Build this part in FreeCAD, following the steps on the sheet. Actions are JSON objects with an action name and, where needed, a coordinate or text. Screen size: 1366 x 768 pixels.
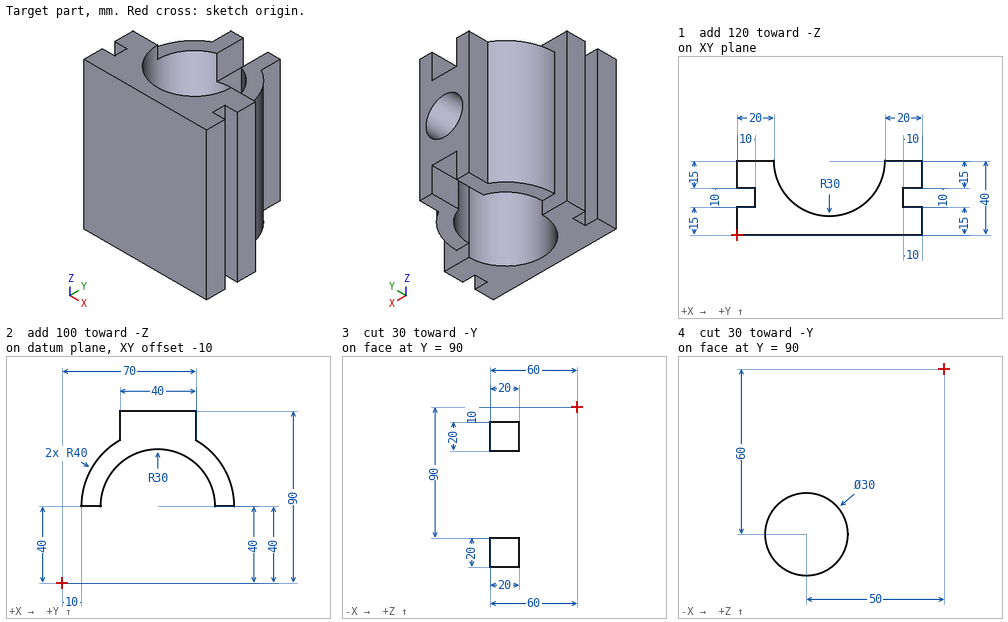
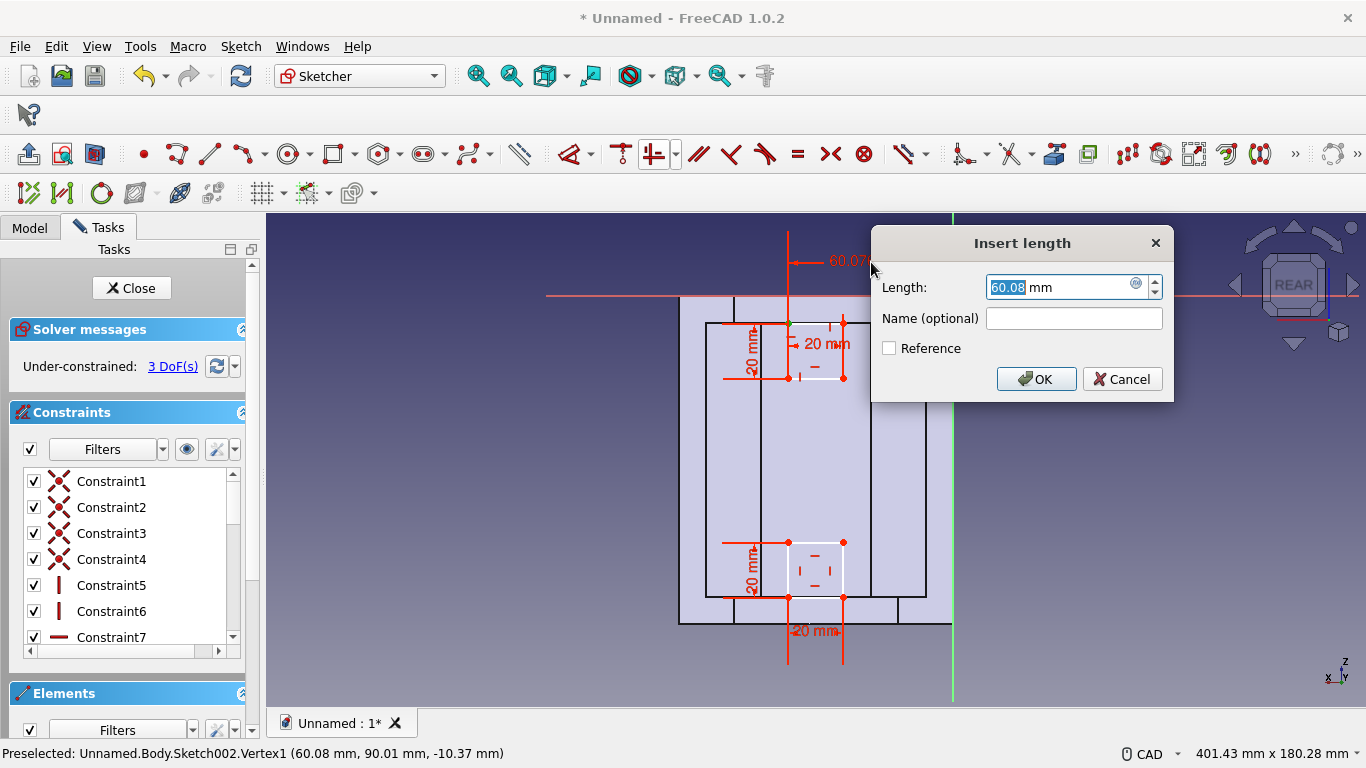
{"action": "type", "text": "60"}
{"action": "key", "text": "Return"}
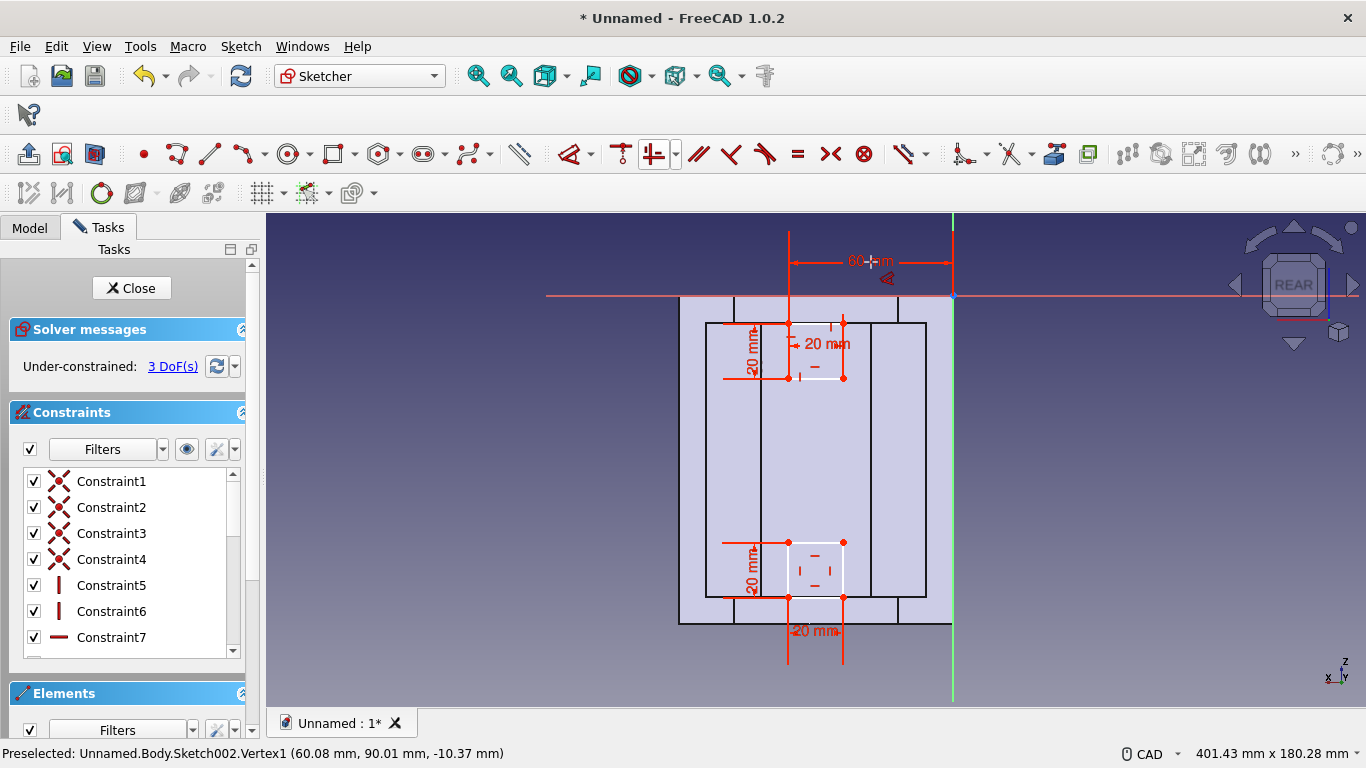
{"action": "scroll", "coordinate": [789, 324], "scroll_direction": "up", "scroll_amount": 2}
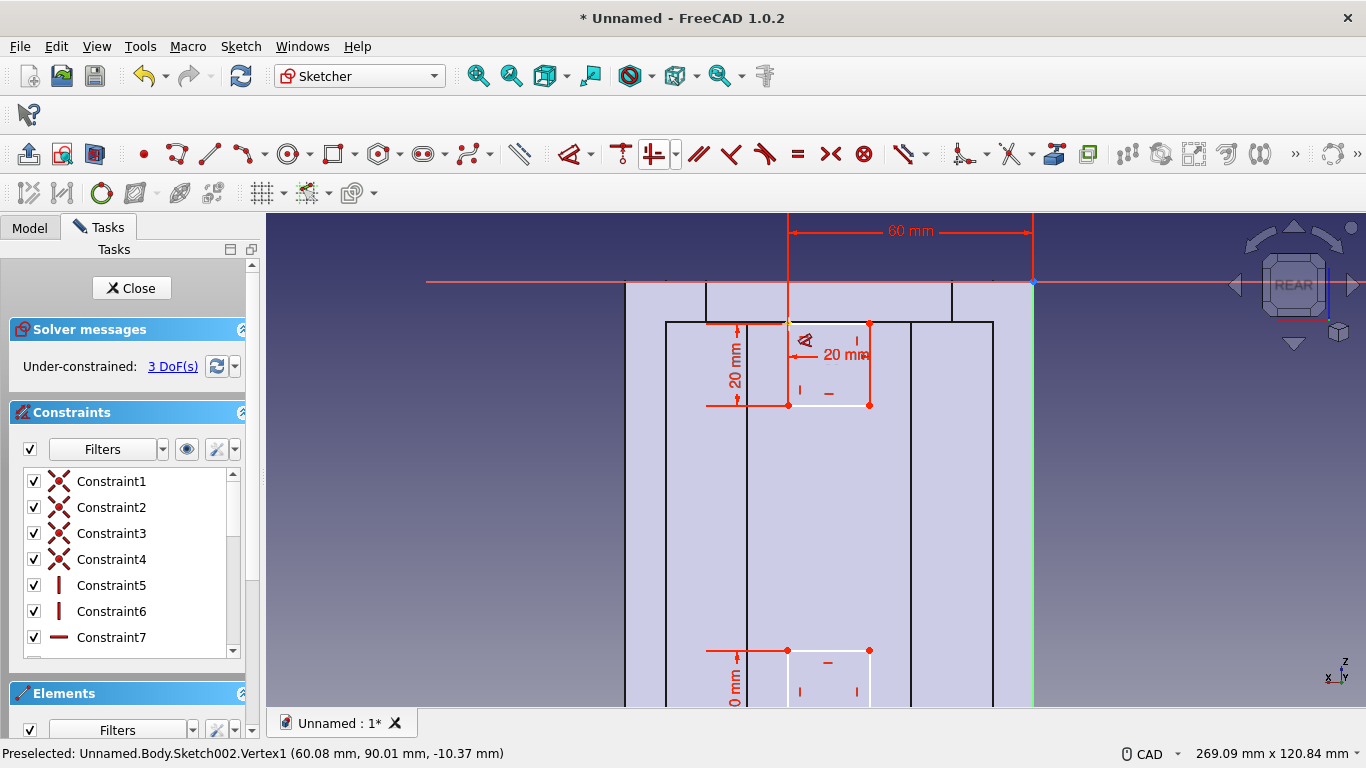
{"action": "left_click", "coordinate": [788, 324]}
{"action": "left_click", "coordinate": [1067, 303]}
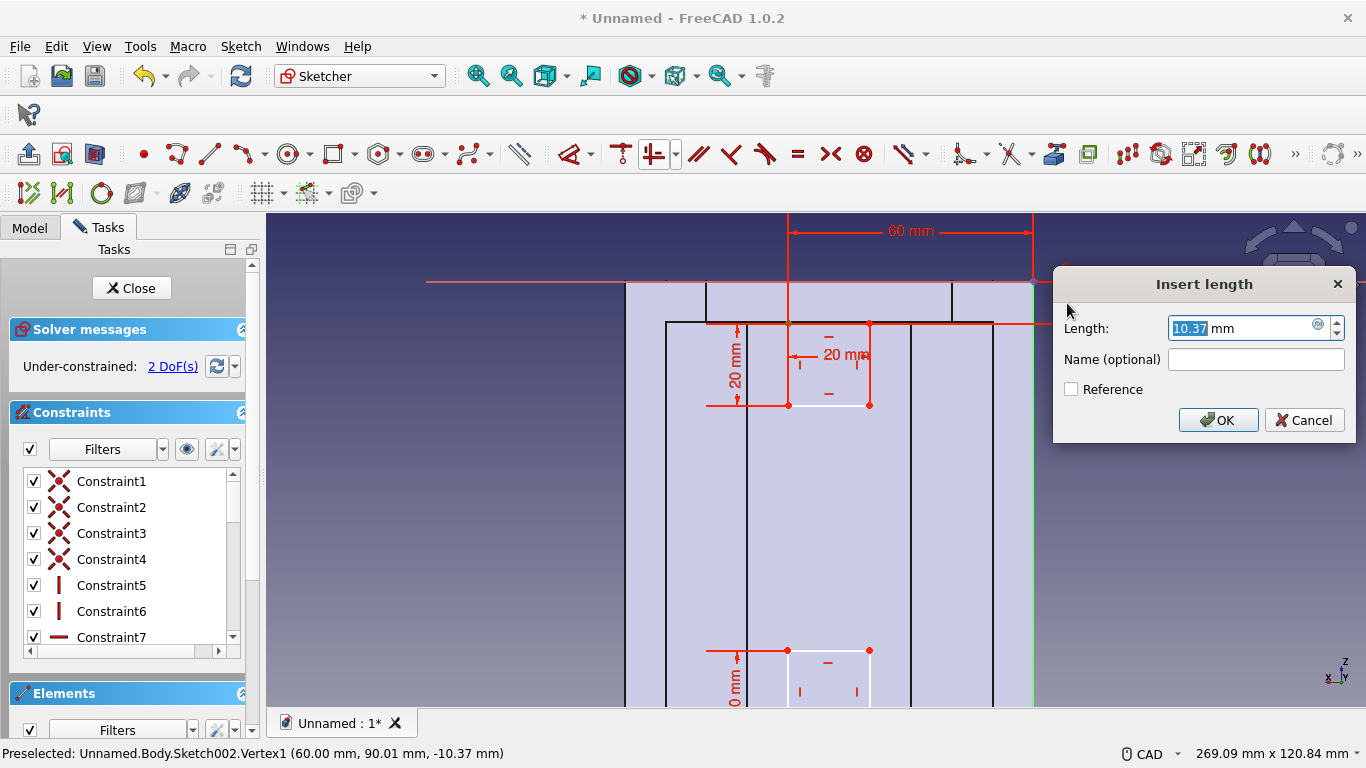
{"action": "type", "text": "10"}
{"action": "key", "text": "Return"}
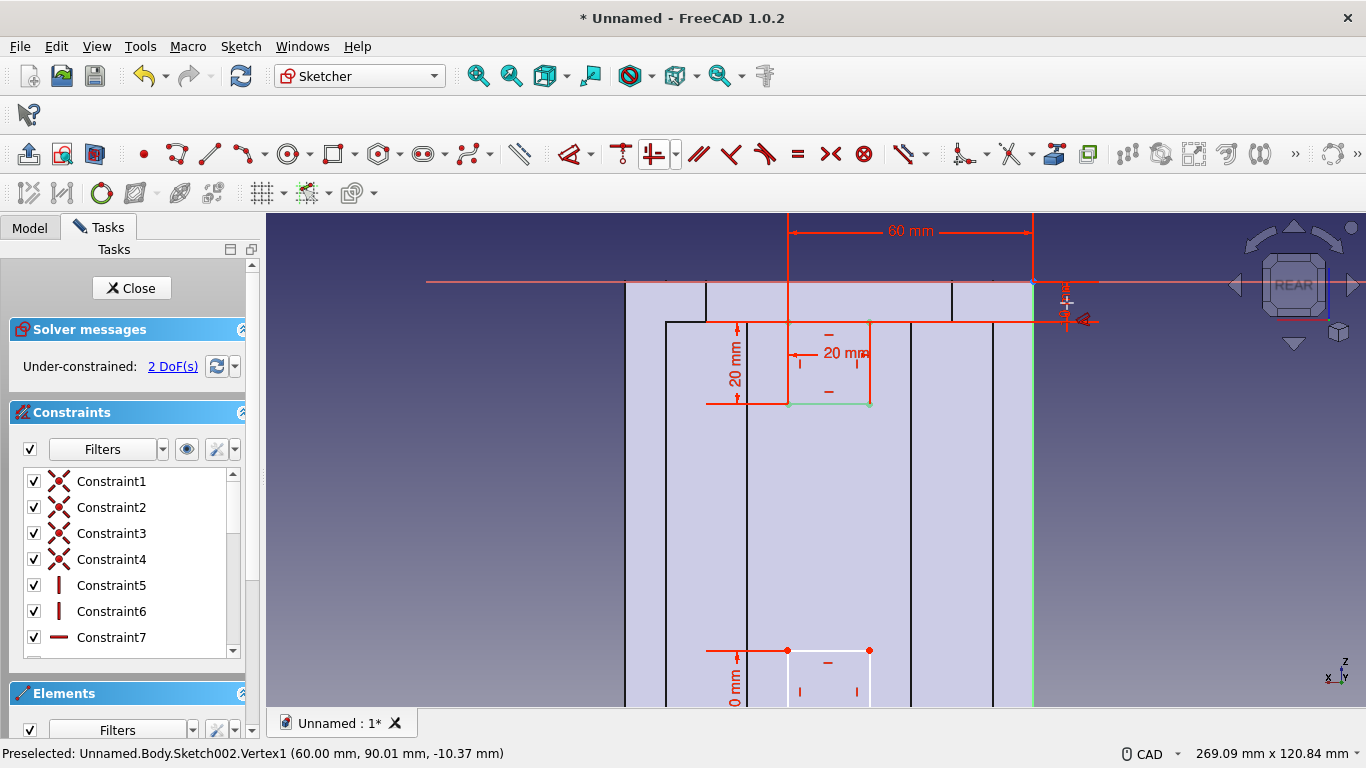
{"action": "left_click", "coordinate": [788, 651]}
{"action": "left_click", "coordinate": [825, 248]}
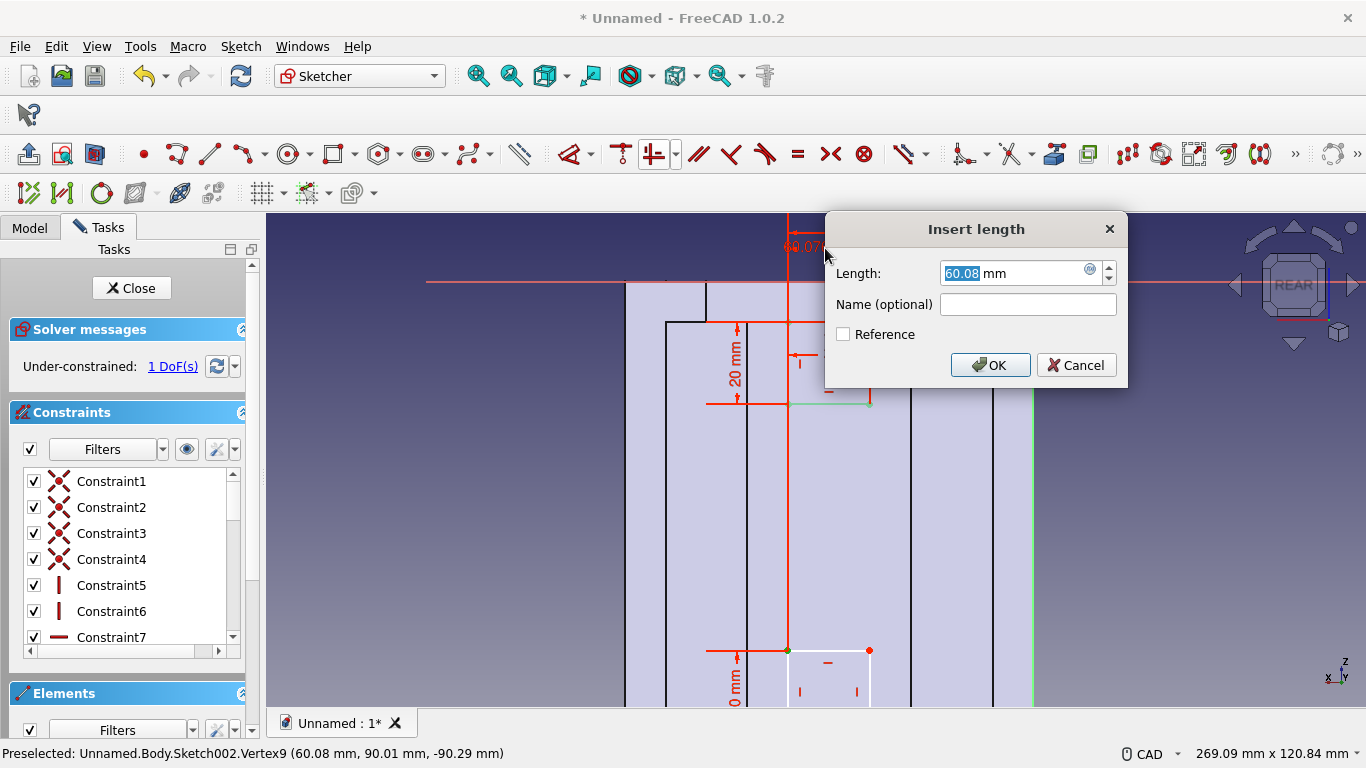
{"action": "type", "text": "60"}
{"action": "key", "text": "Return"}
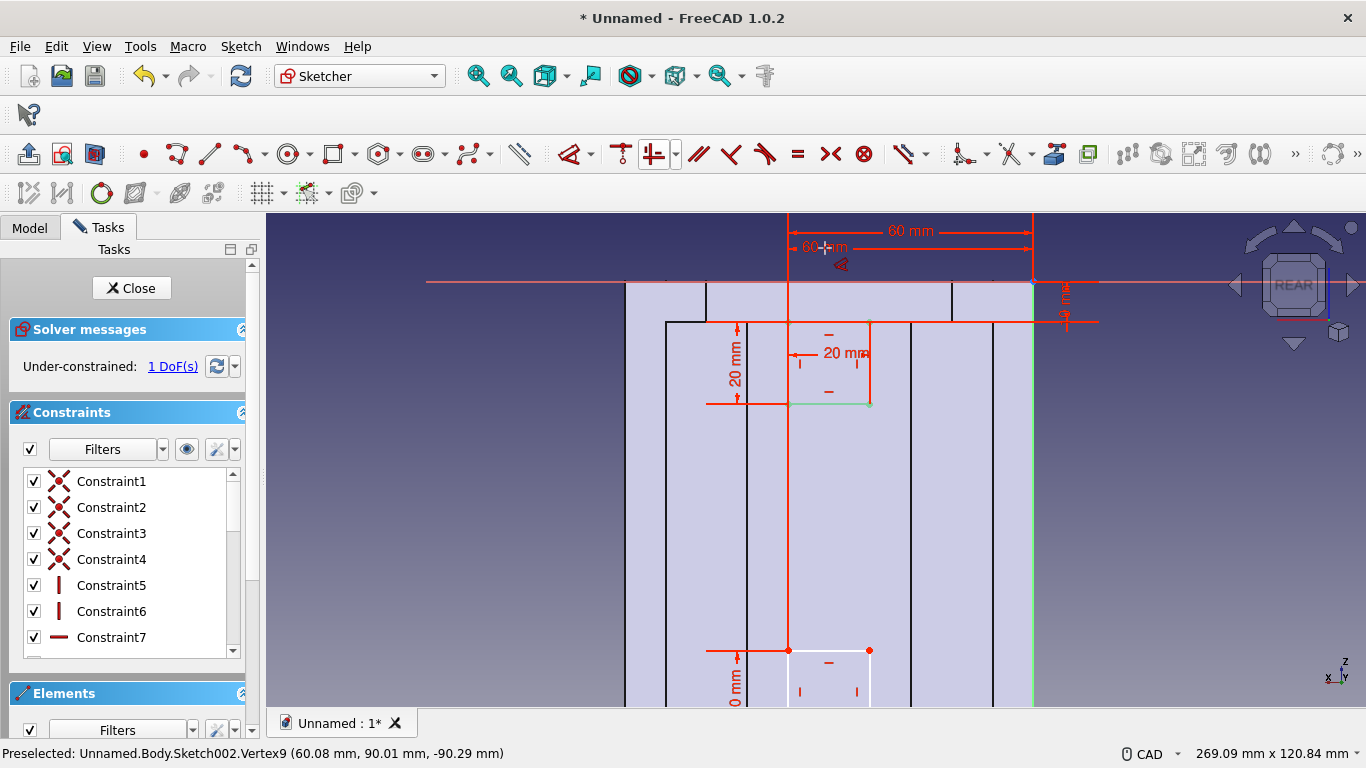
{"action": "left_click", "coordinate": [788, 651]}
{"action": "left_click", "coordinate": [1067, 466]}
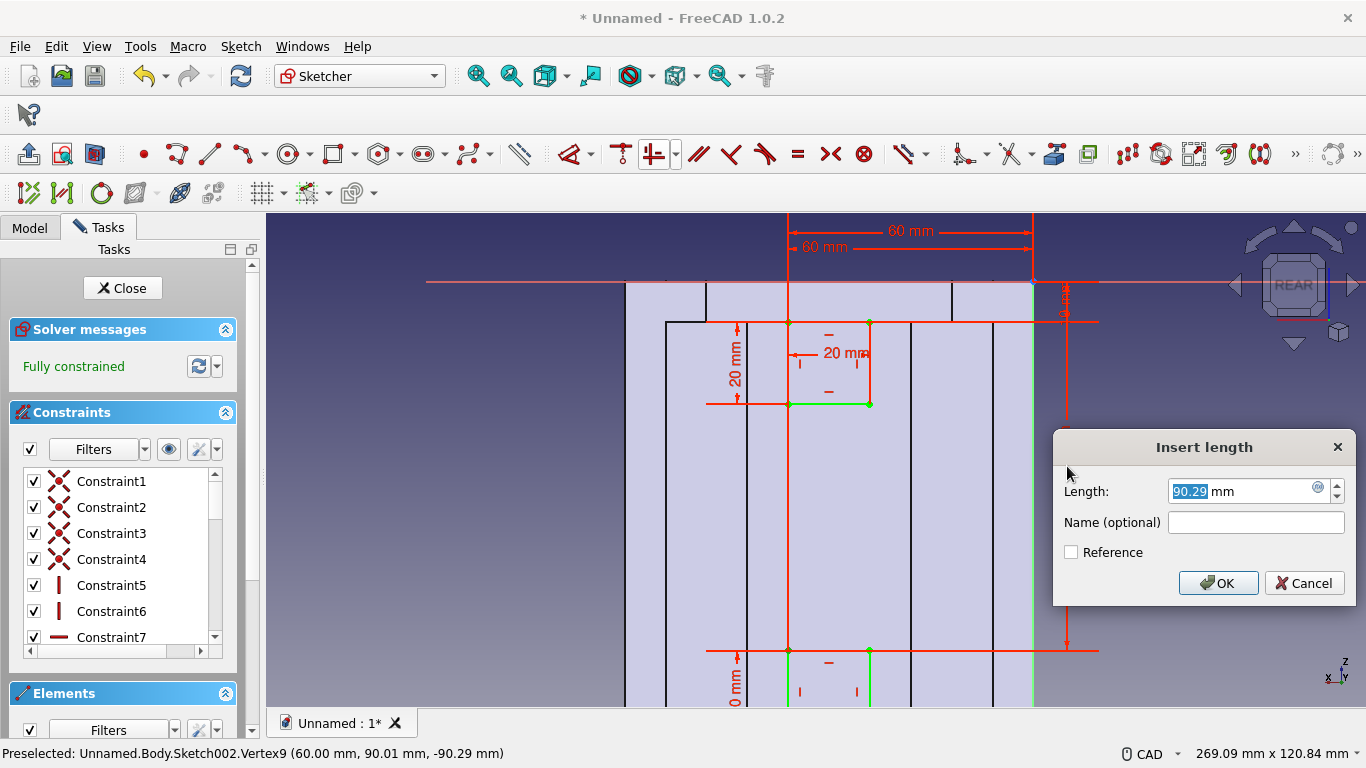
{"action": "type", "text": "90"}
{"action": "key", "text": "Return"}
{"action": "key", "text": "Escape"}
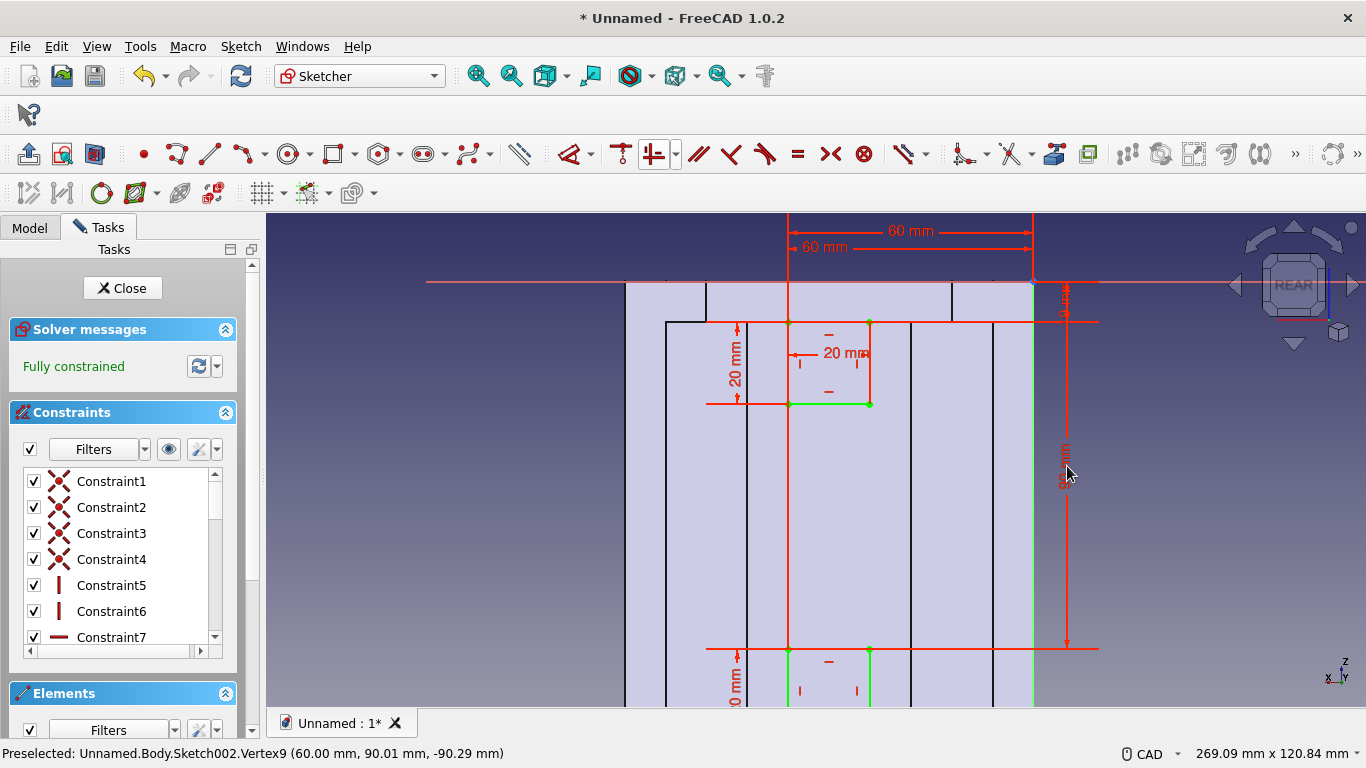
{"action": "left_click", "coordinate": [123, 288]}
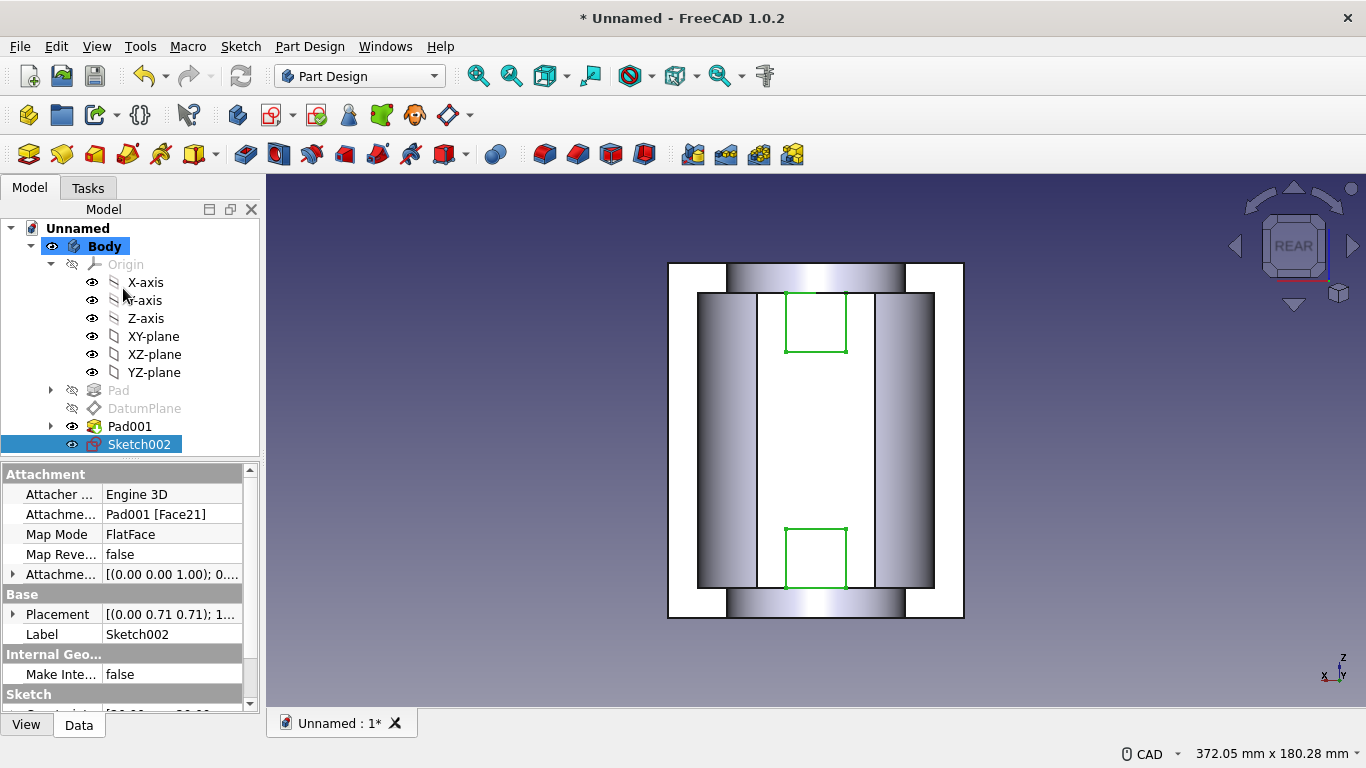
{"action": "left_click", "coordinate": [246, 154]}